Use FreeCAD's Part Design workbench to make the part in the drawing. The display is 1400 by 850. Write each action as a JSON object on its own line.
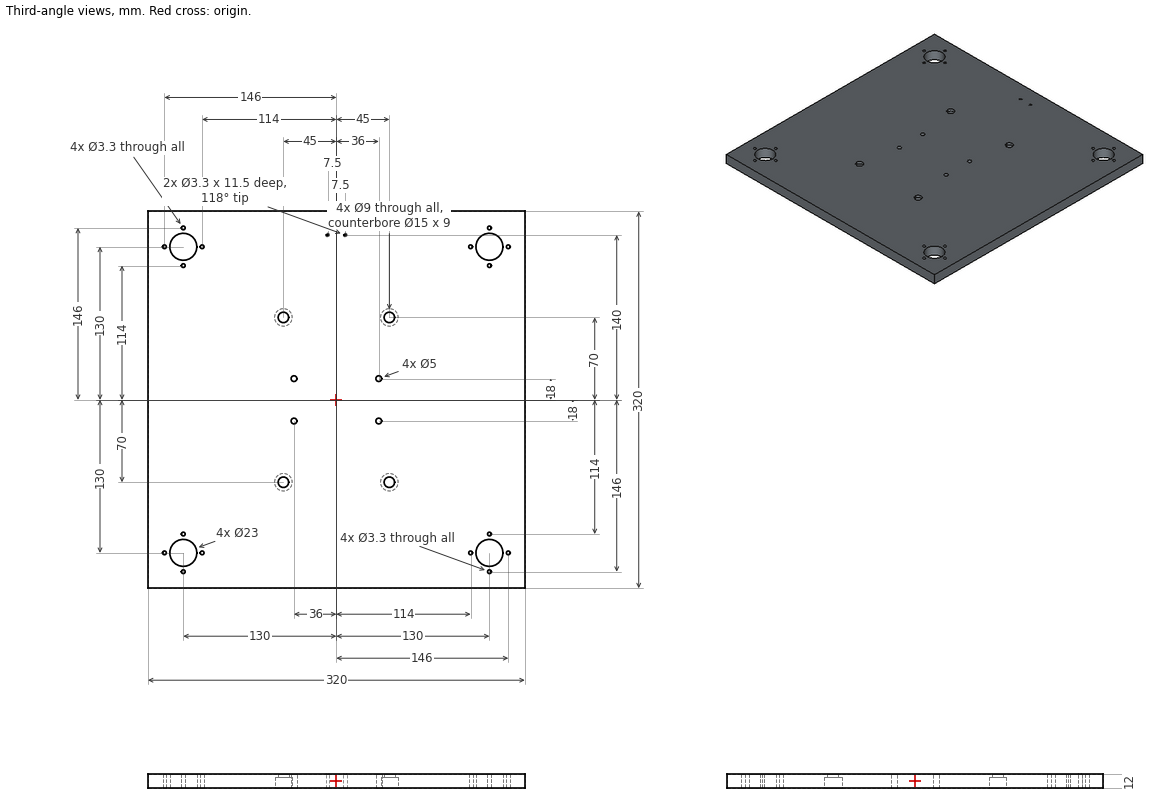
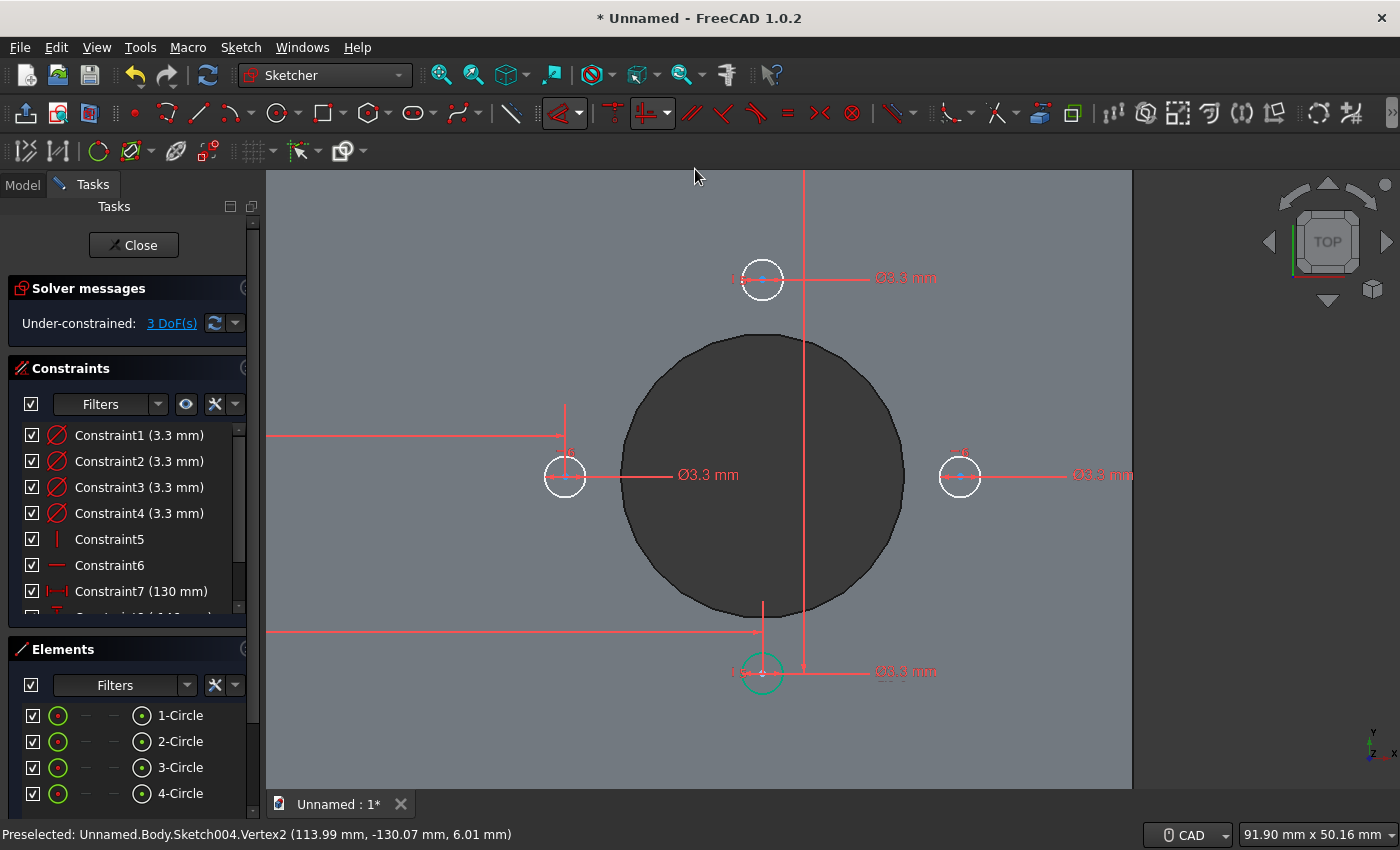
{"action": "left_click", "coordinate": [565, 477]}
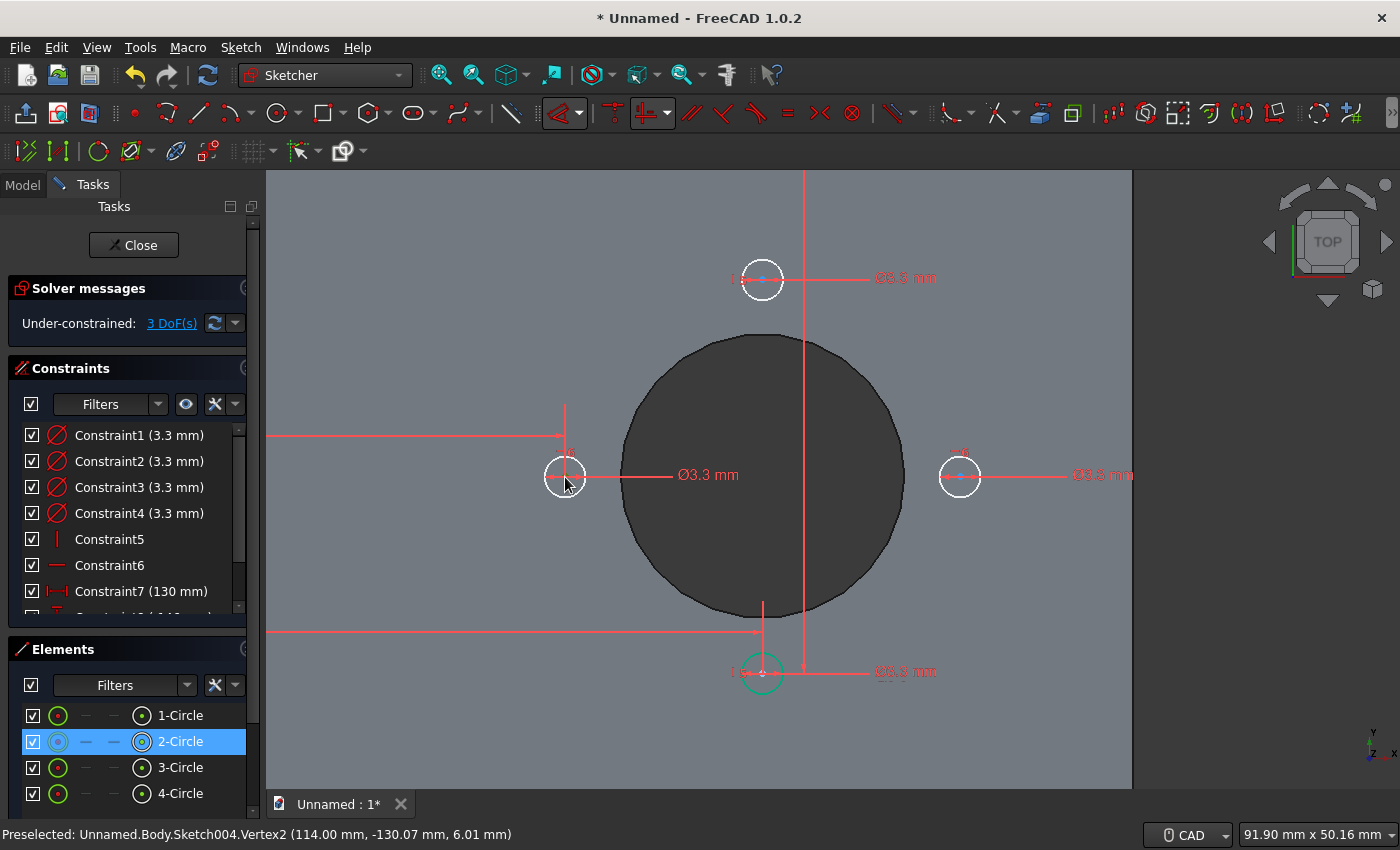
{"action": "left_click", "coordinate": [582, 114]}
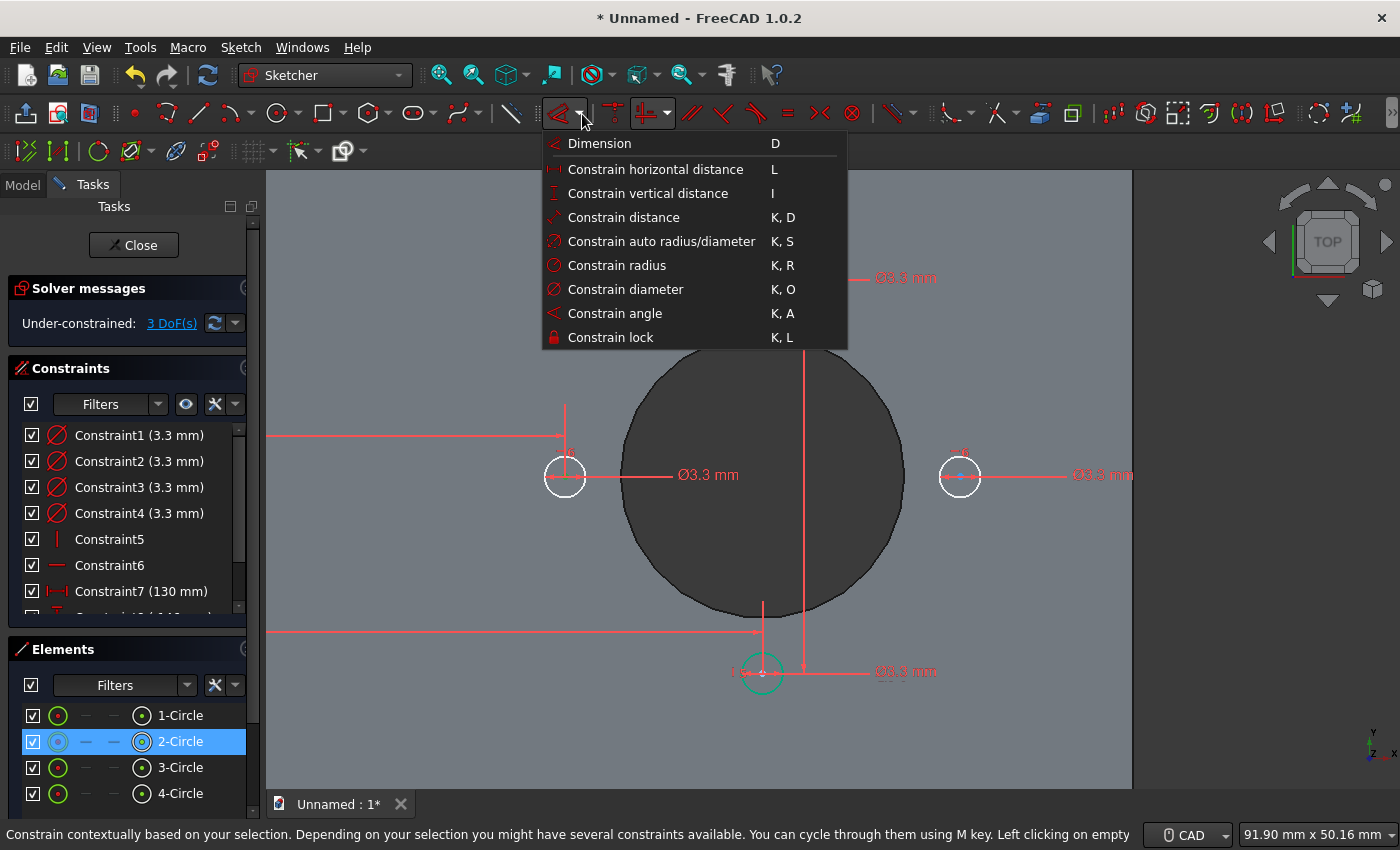
{"action": "left_click", "coordinate": [695, 193]}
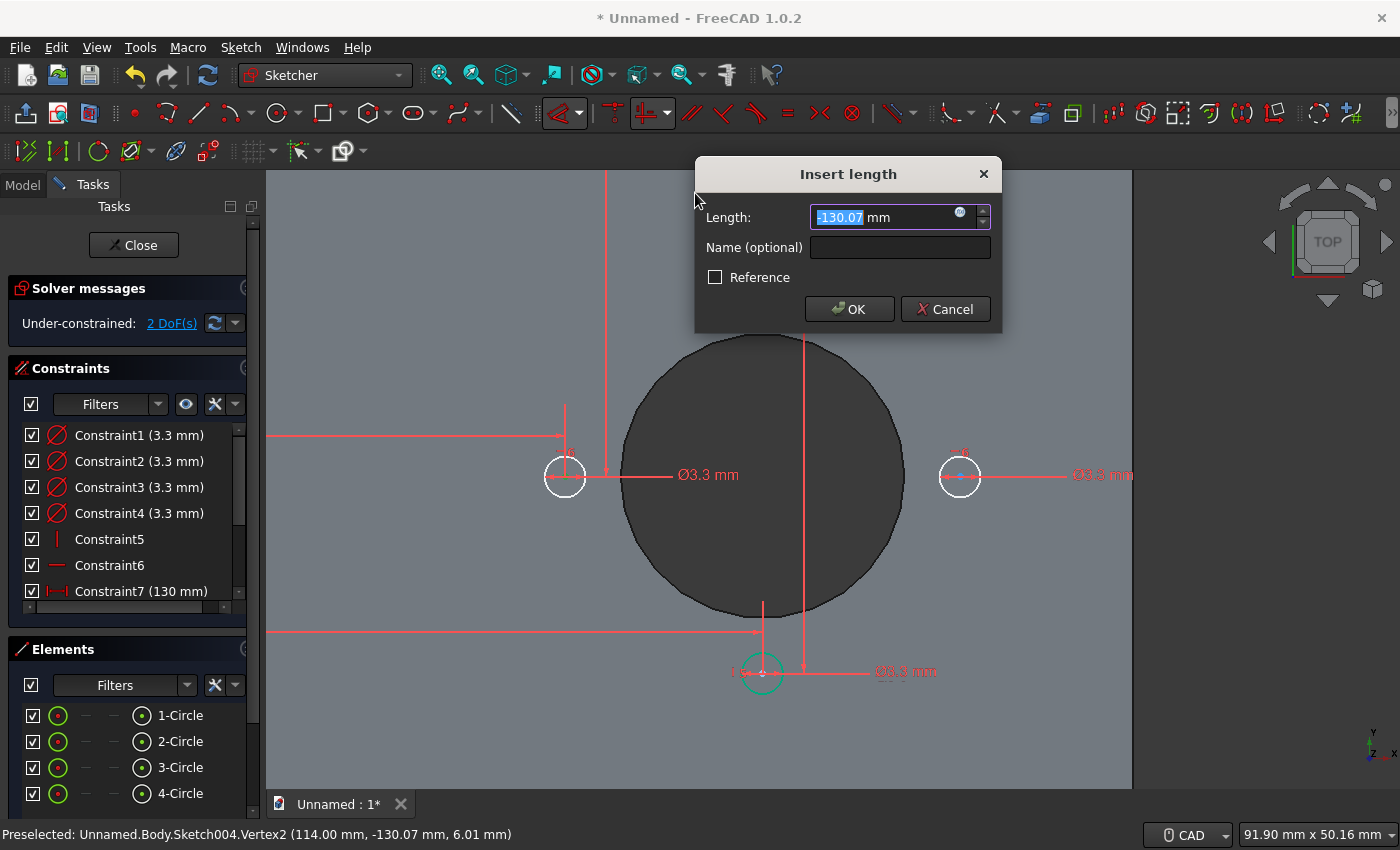
{"action": "type", "text": "-130"}
{"action": "key", "text": "Return"}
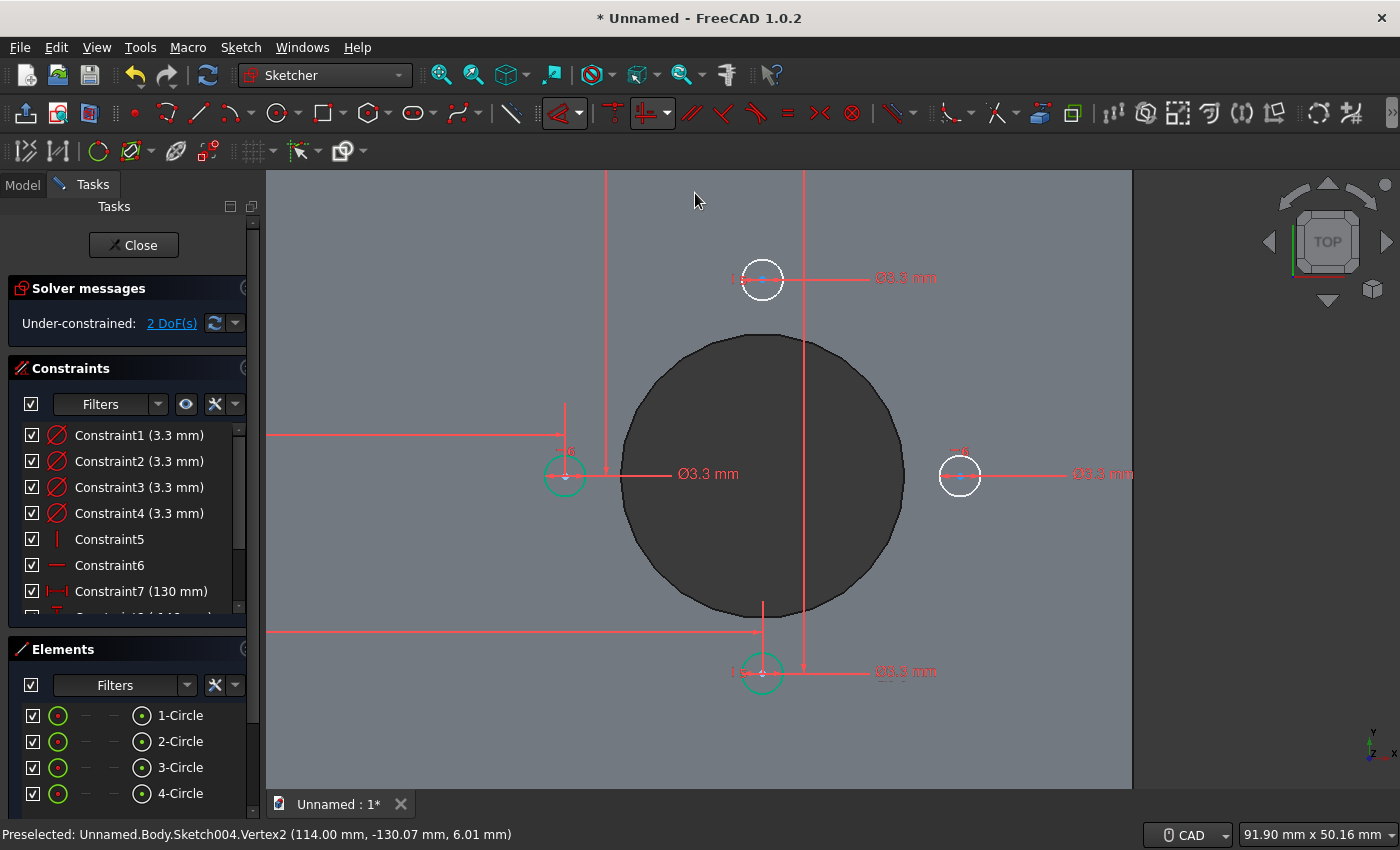
{"action": "left_click", "coordinate": [763, 280]}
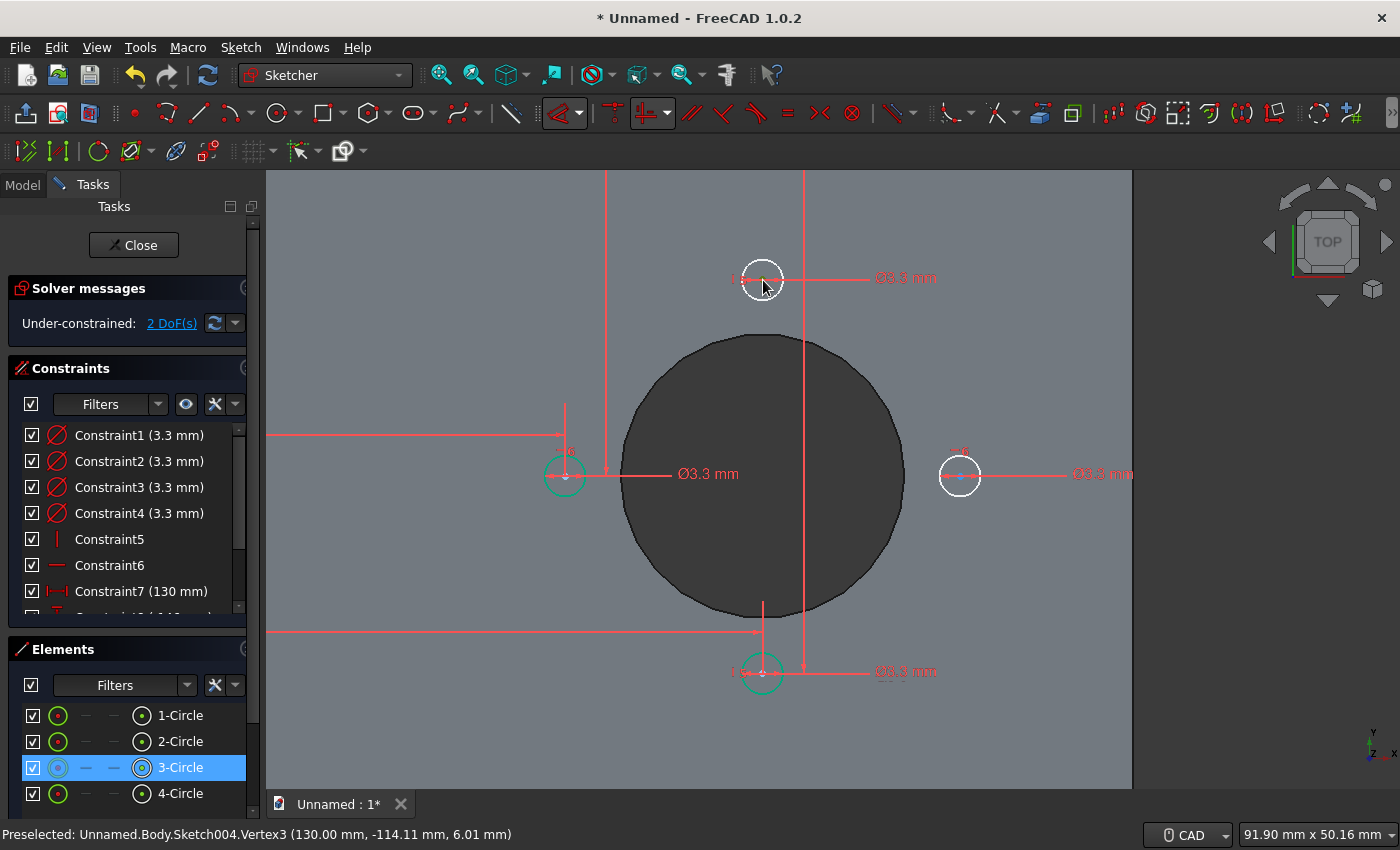
{"action": "left_click", "coordinate": [582, 114]}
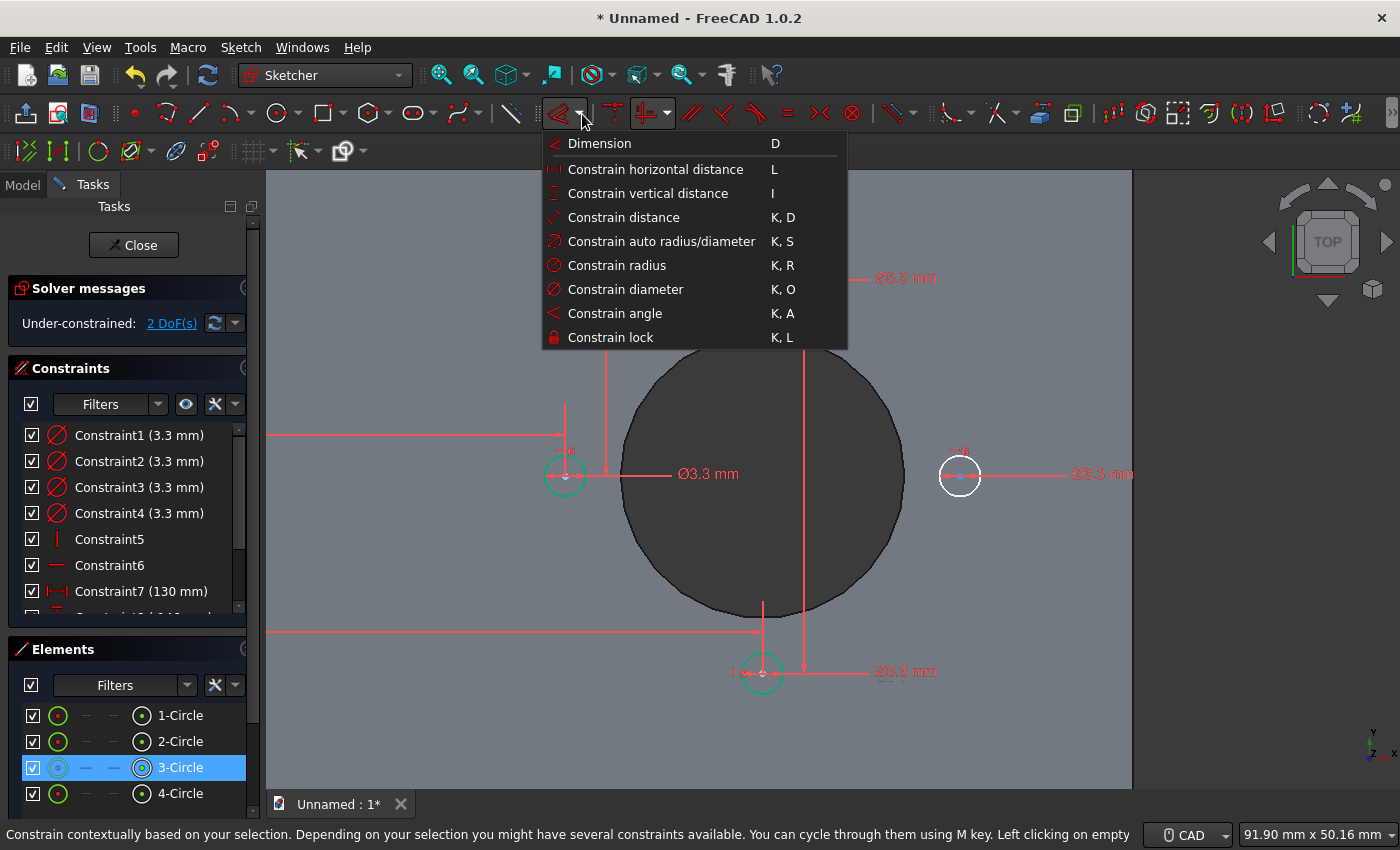
{"action": "left_click", "coordinate": [695, 193]}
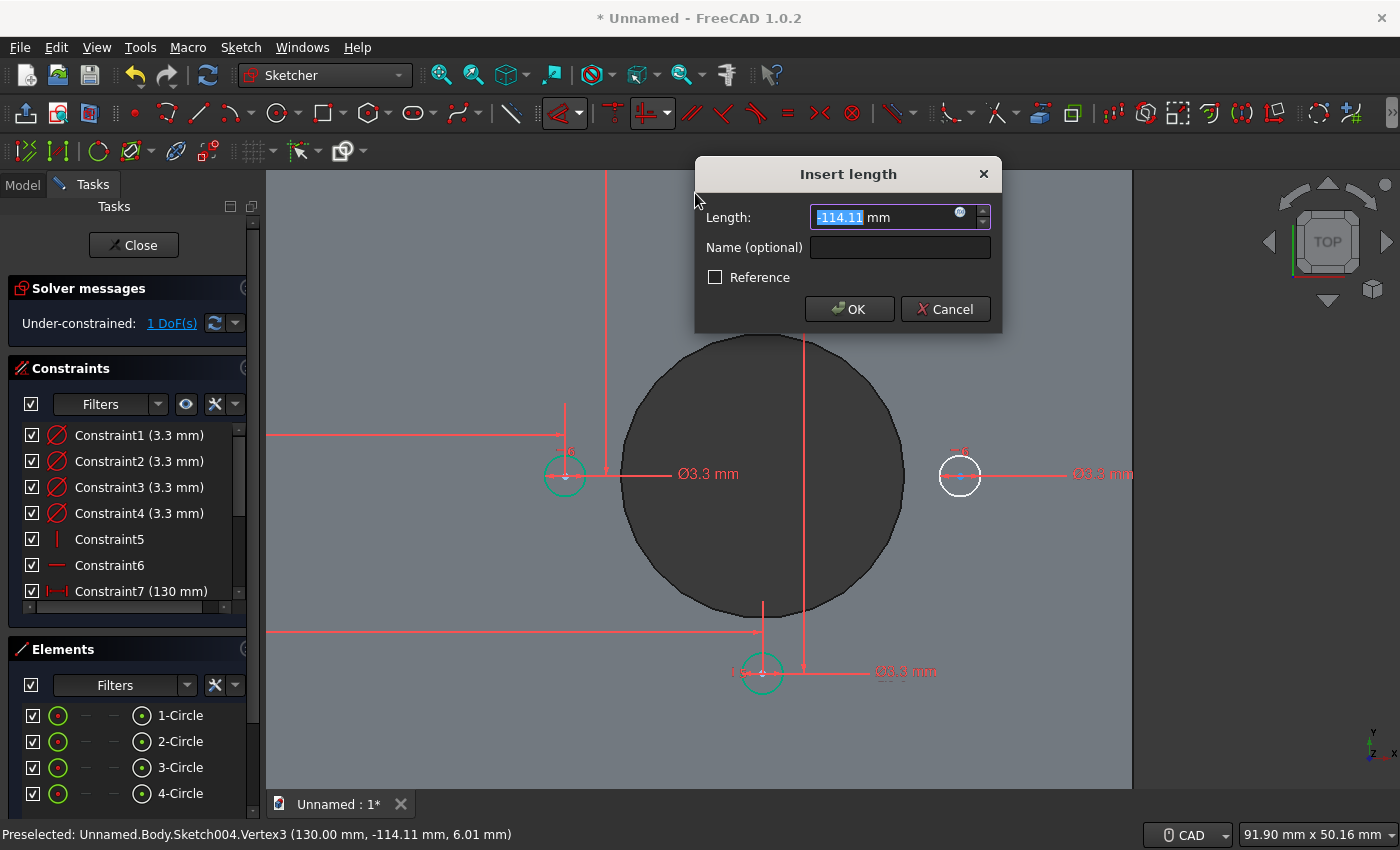
{"action": "type", "text": "-114"}
{"action": "key", "text": "Return"}